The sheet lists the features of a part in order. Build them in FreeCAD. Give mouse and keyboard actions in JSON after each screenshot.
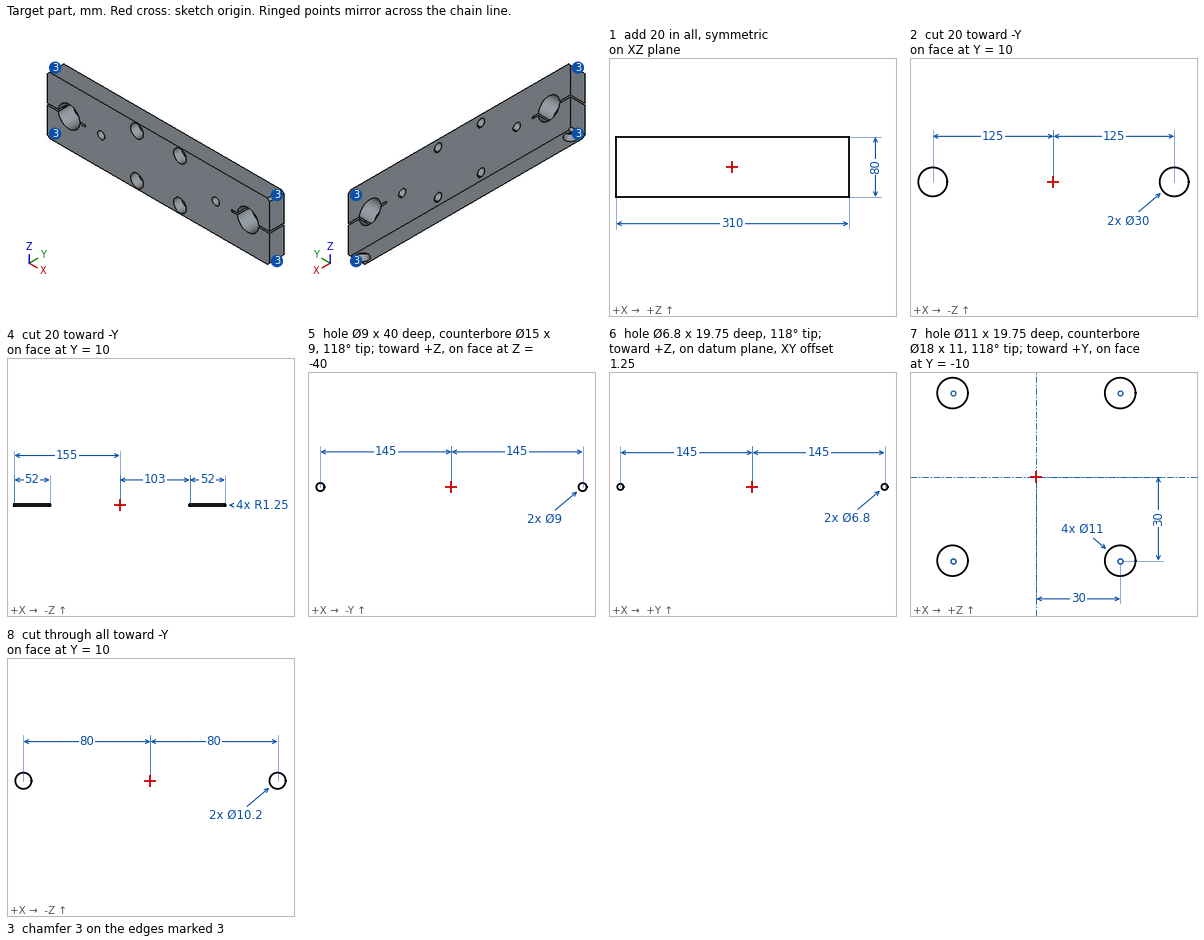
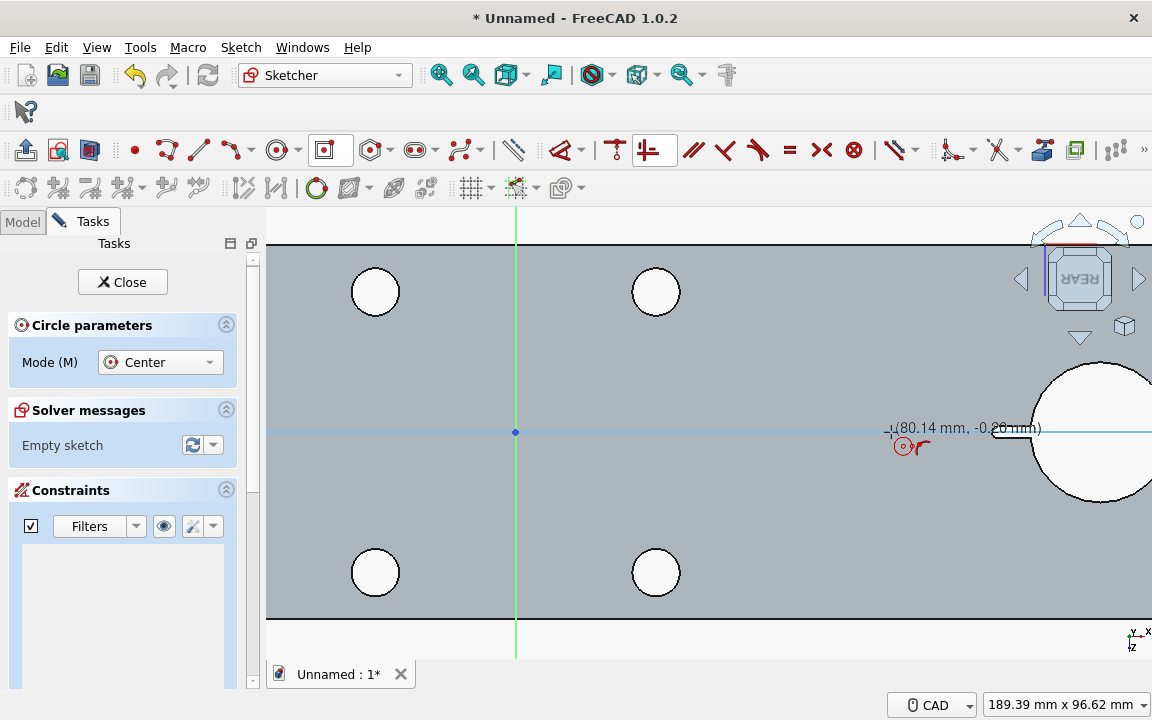
{"action": "left_click", "coordinate": [890, 432]}
{"action": "mouse_move", "coordinate": [907, 415]}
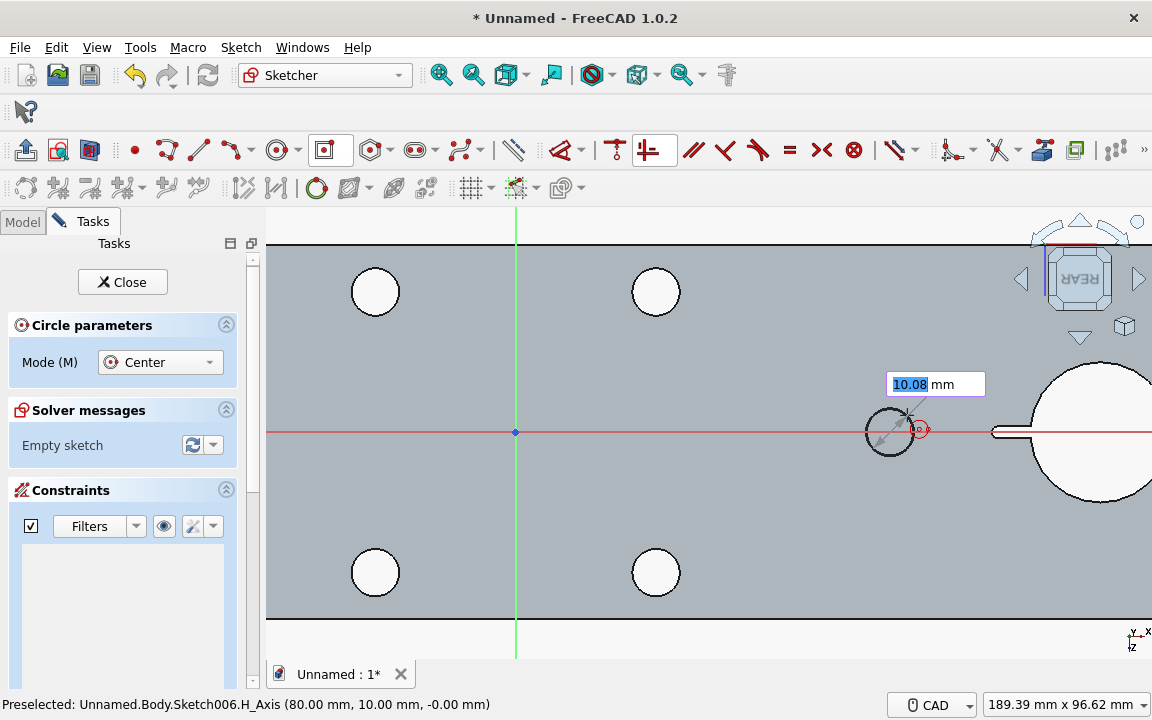
{"action": "type", "text": "10.2"}
{"action": "key", "text": "Return"}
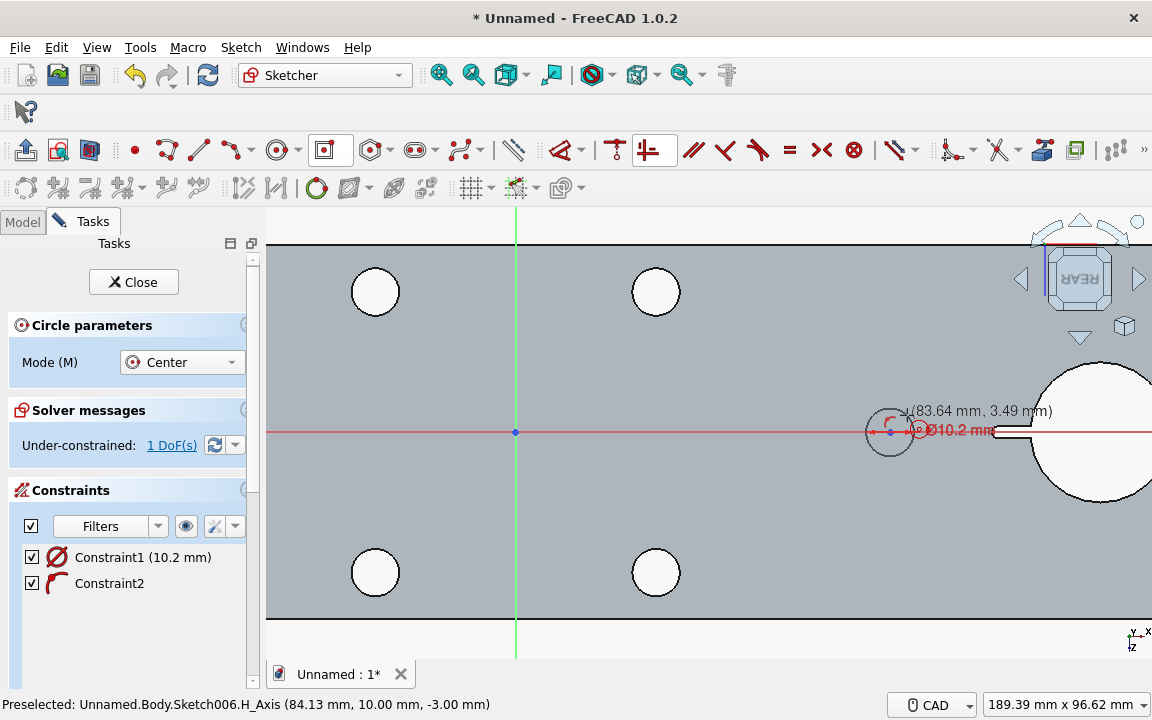
{"action": "scroll", "coordinate": [894, 434], "scroll_direction": "down", "scroll_amount": 2}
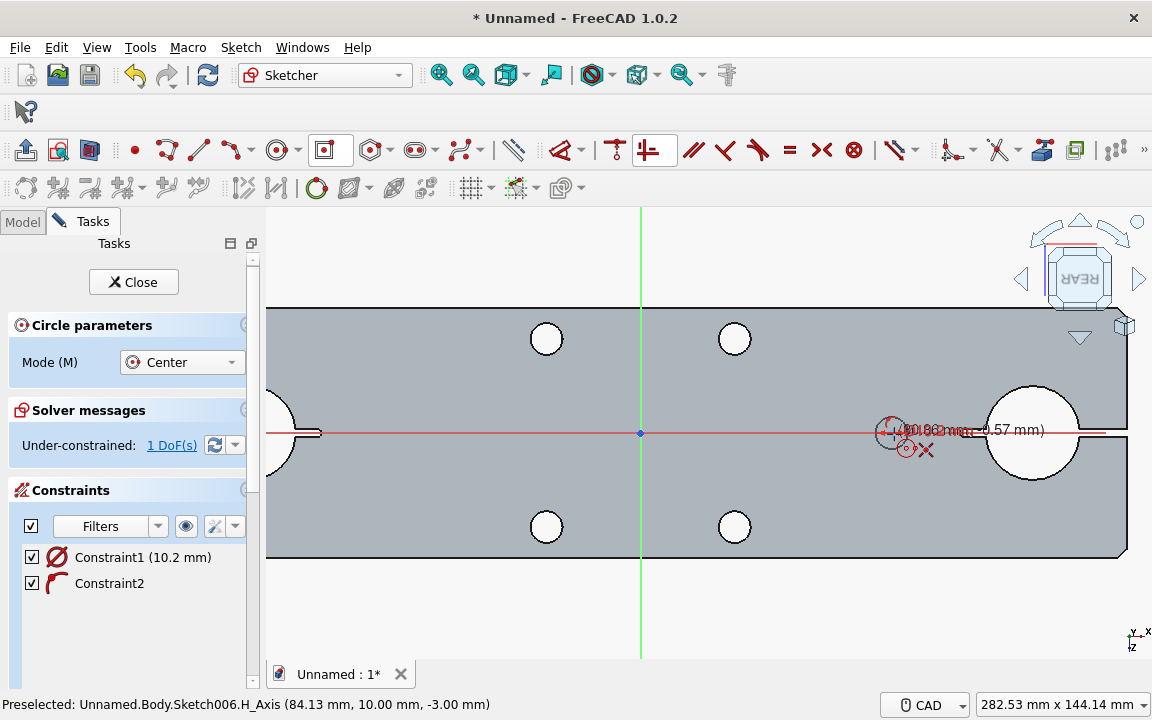
{"action": "scroll", "coordinate": [390, 433], "scroll_direction": "up", "scroll_amount": 2}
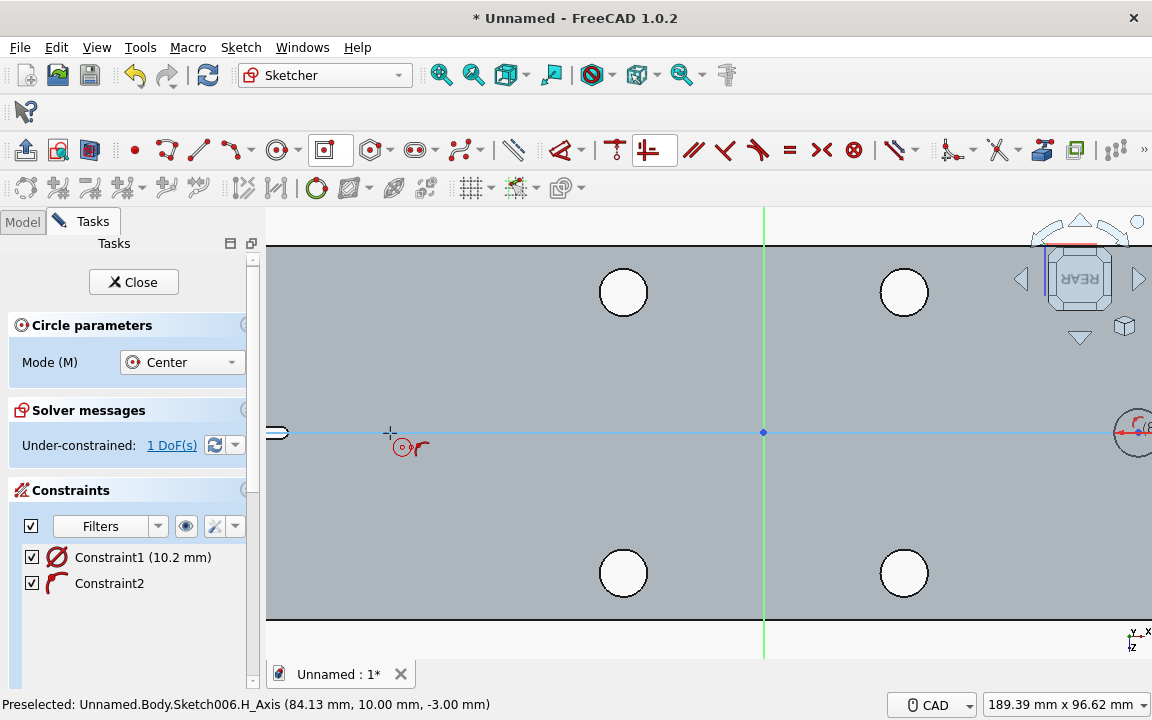
{"action": "left_click", "coordinate": [390, 433]}
{"action": "mouse_move", "coordinate": [406, 416]}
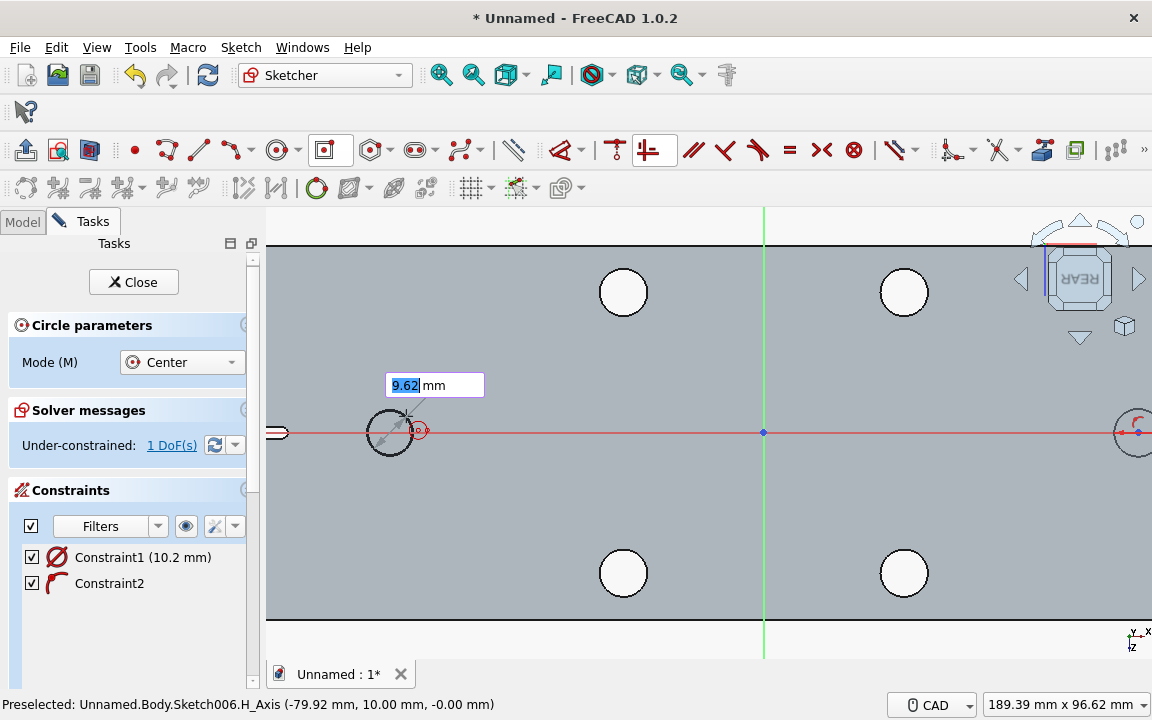
{"action": "type", "text": "10.2"}
{"action": "key", "text": "Return"}
{"action": "key", "text": "Escape"}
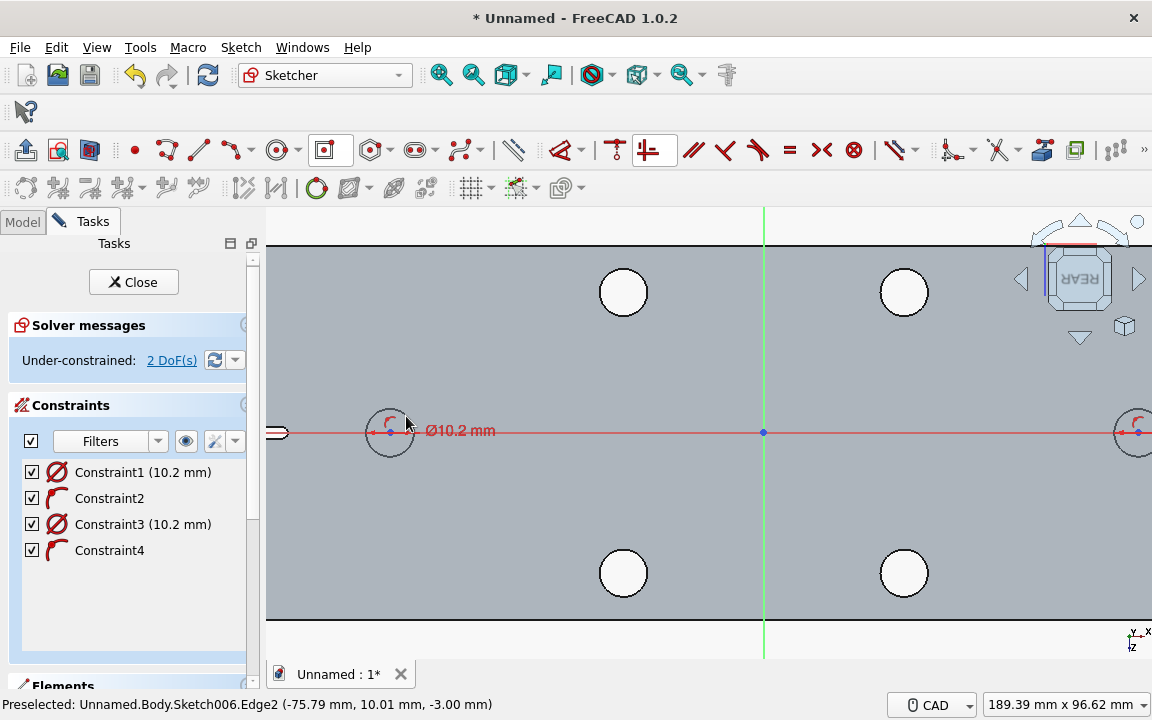
{"action": "left_click", "coordinate": [560, 150]}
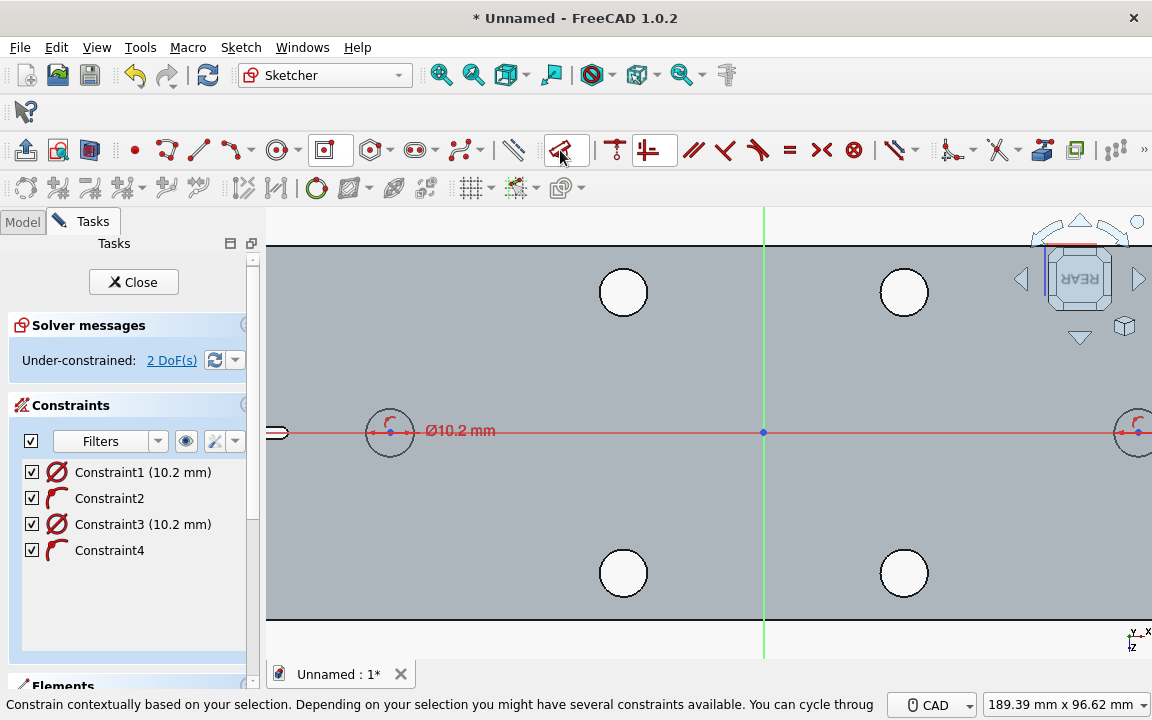
{"action": "scroll", "coordinate": [390, 433], "scroll_direction": "down", "scroll_amount": 2}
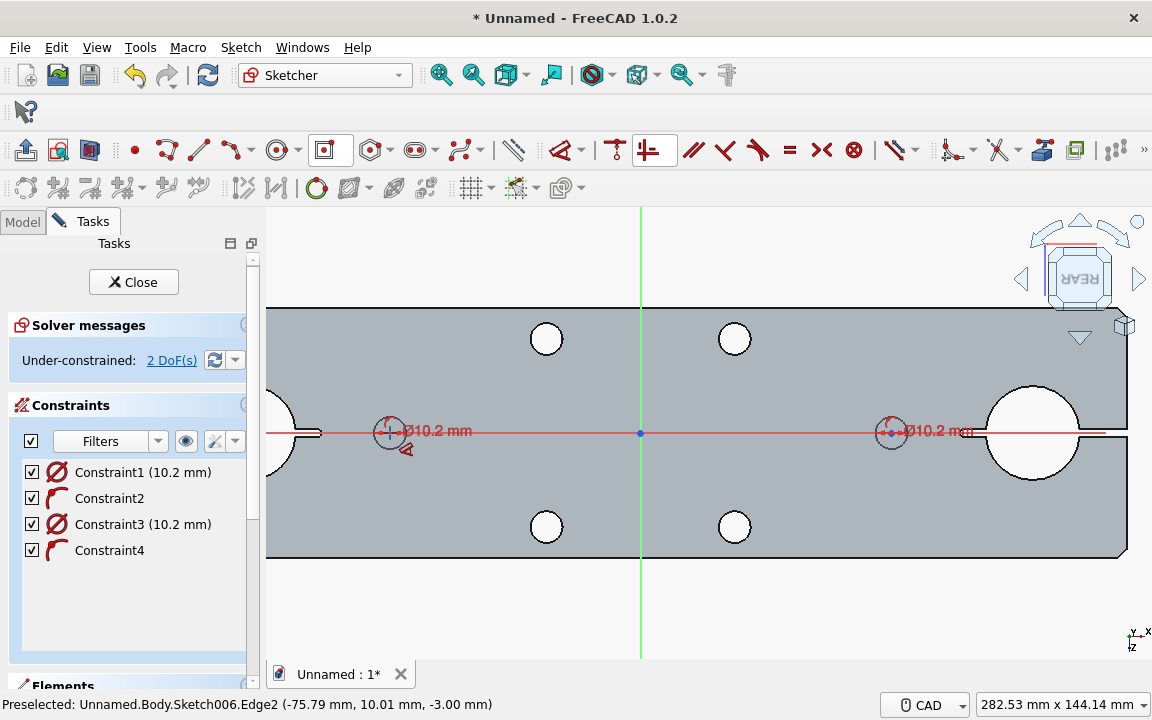
{"action": "left_click", "coordinate": [892, 433]}
{"action": "left_click", "coordinate": [766, 467]}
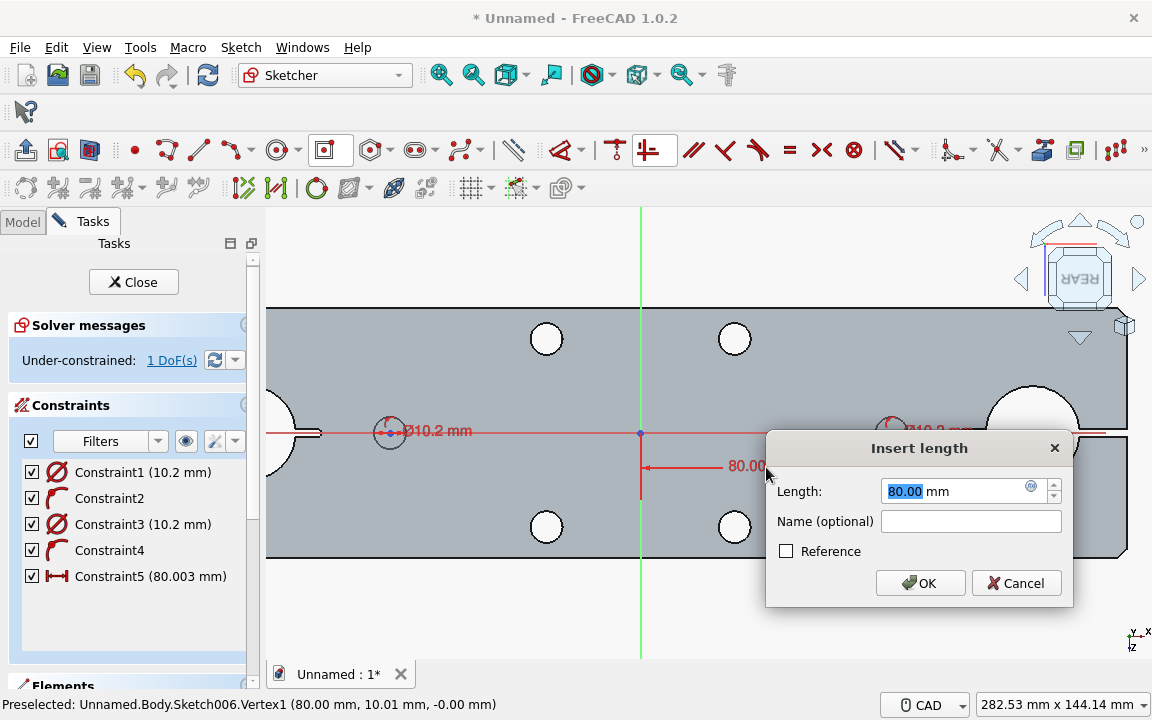
{"action": "type", "text": "80"}
{"action": "key", "text": "Return"}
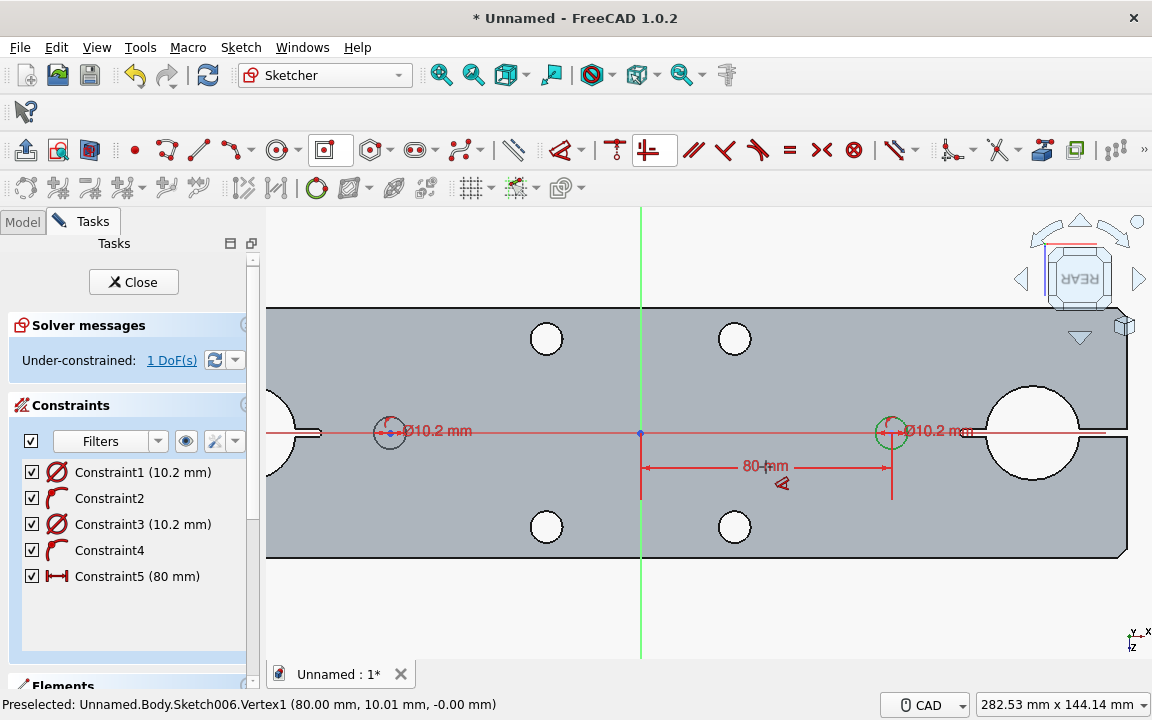
{"action": "left_click", "coordinate": [390, 433]}
{"action": "left_click", "coordinate": [515, 467]}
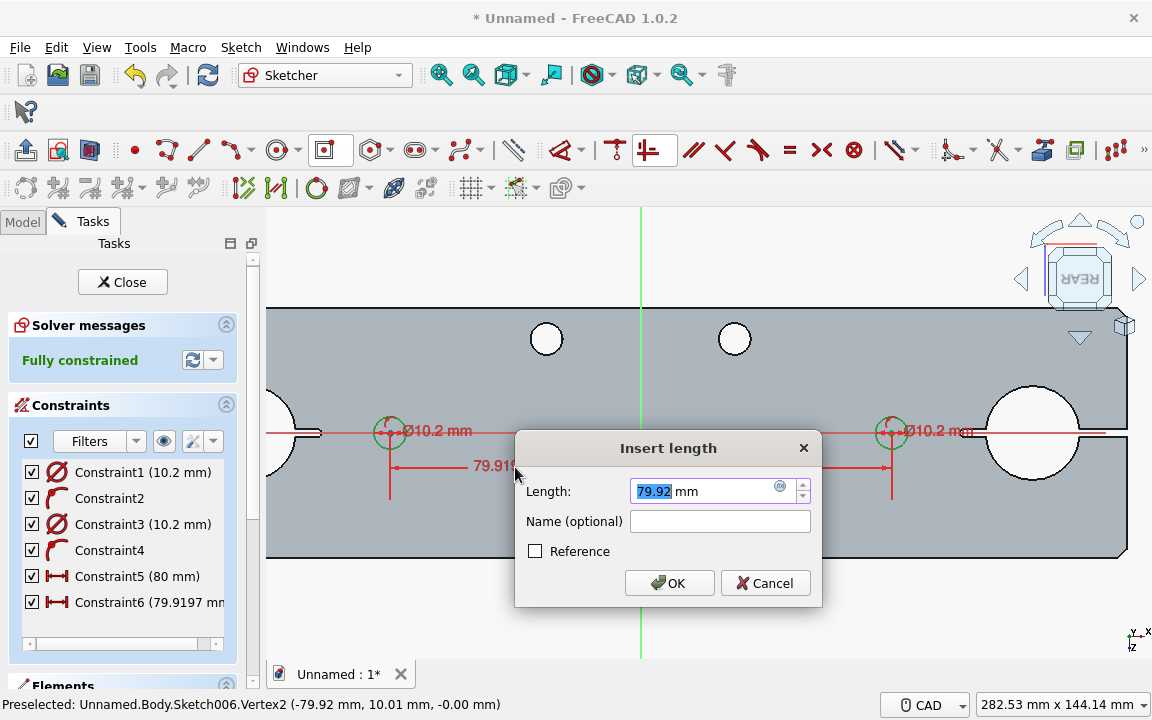
{"action": "type", "text": "80"}
{"action": "key", "text": "Return"}
{"action": "key", "text": "Escape"}